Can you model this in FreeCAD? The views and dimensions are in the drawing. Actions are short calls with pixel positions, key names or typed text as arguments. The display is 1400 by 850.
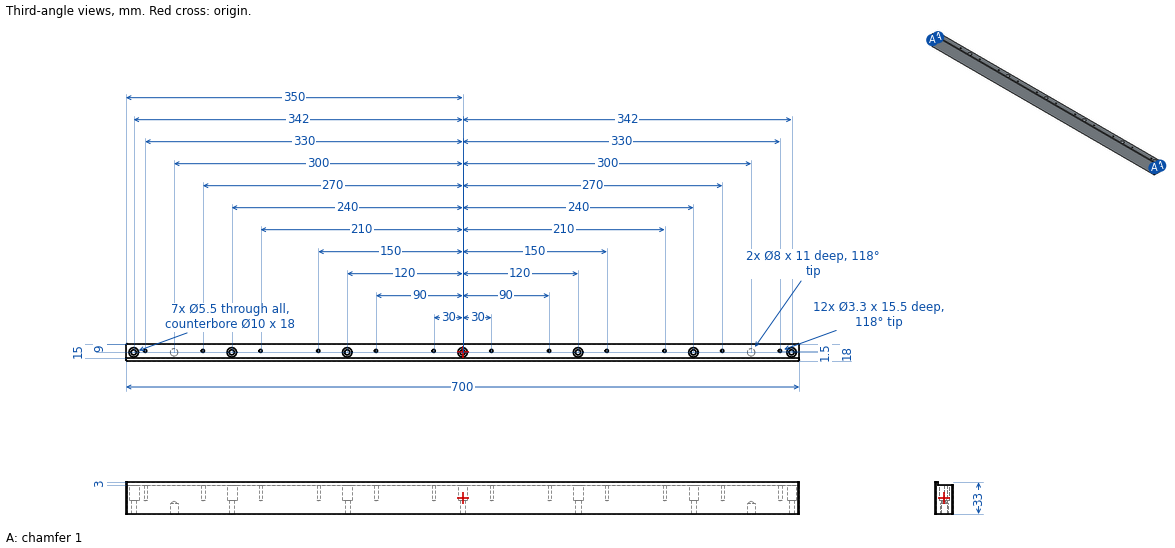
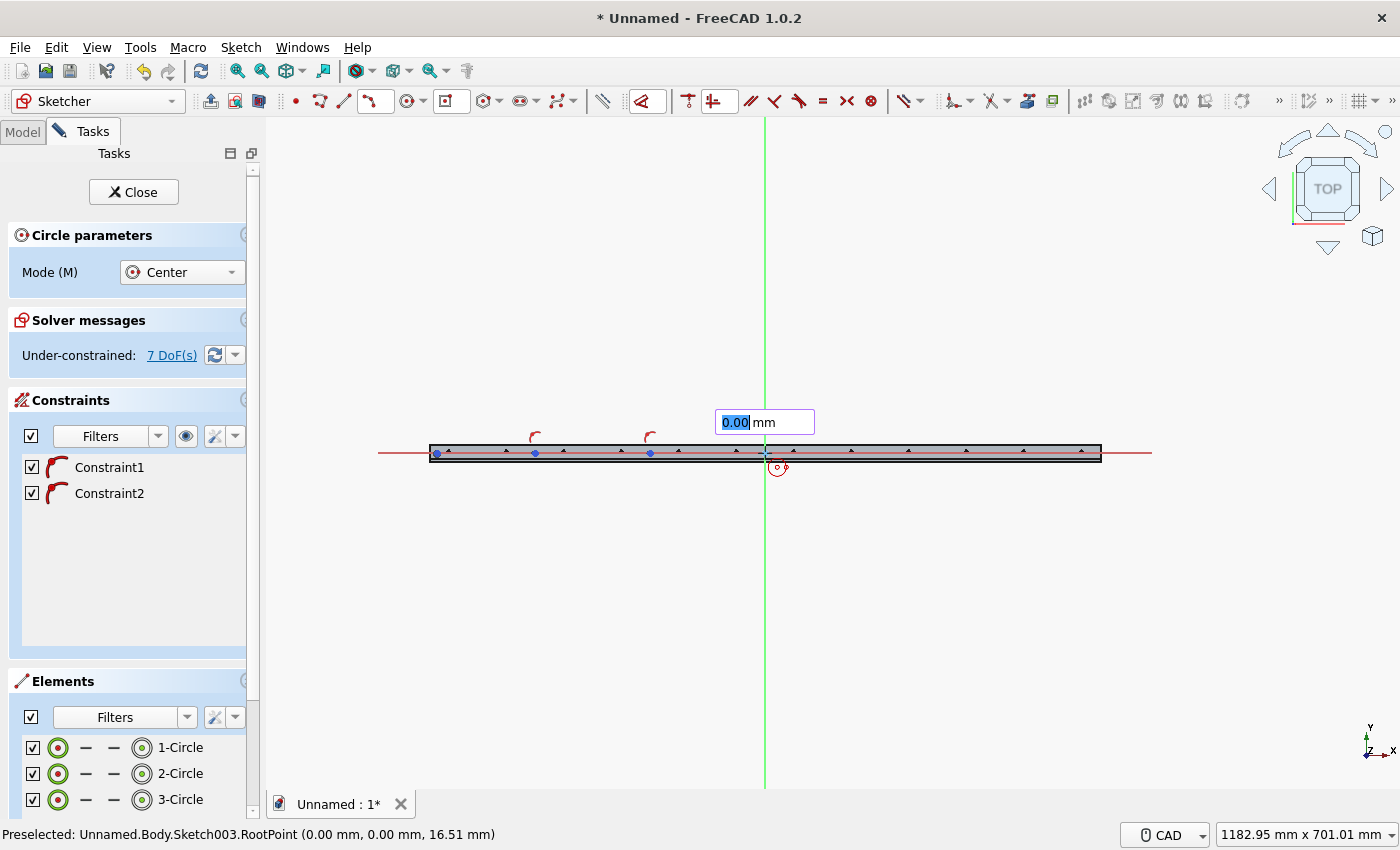
scroll(767, 451, up, 11)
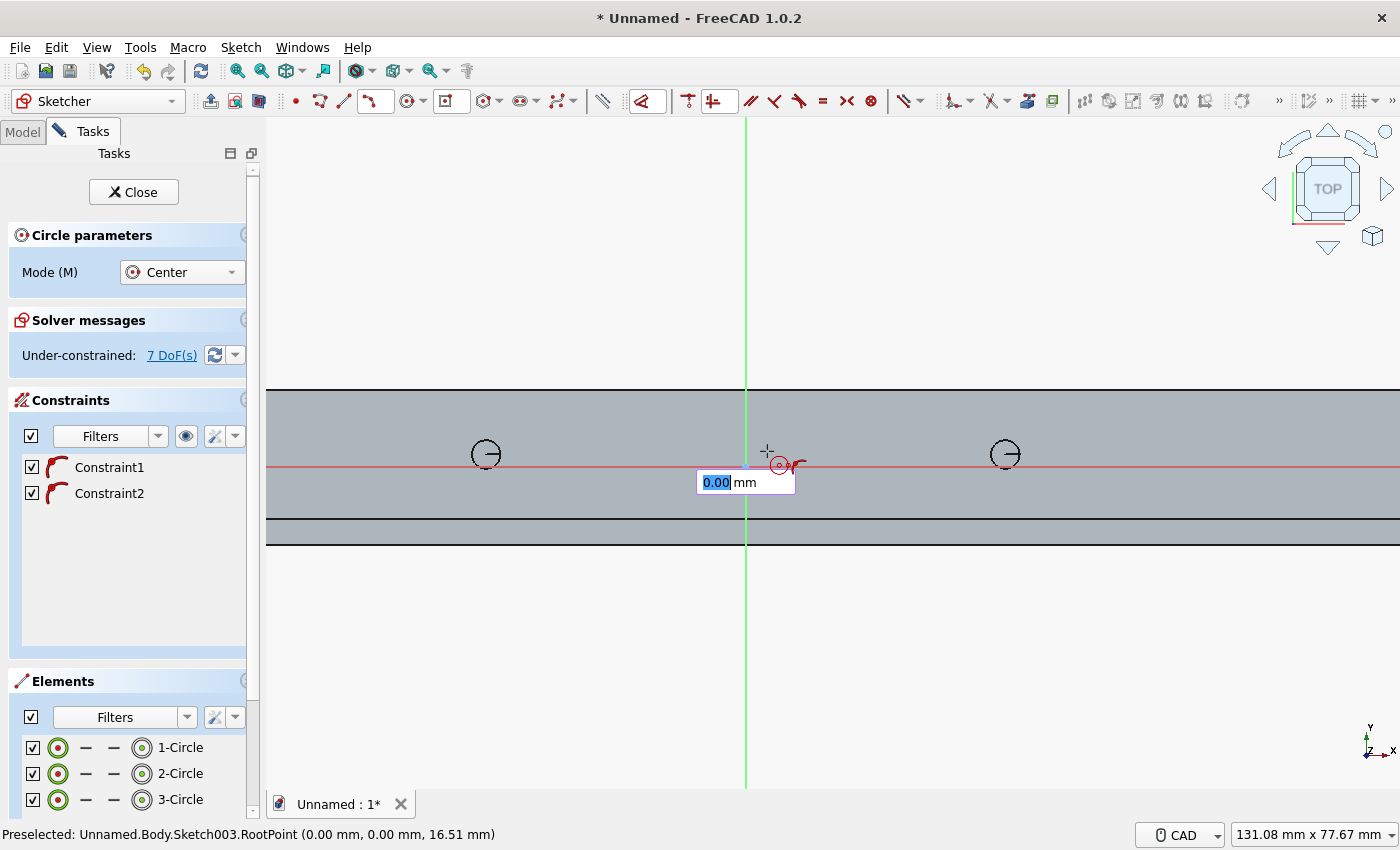
click(763, 451)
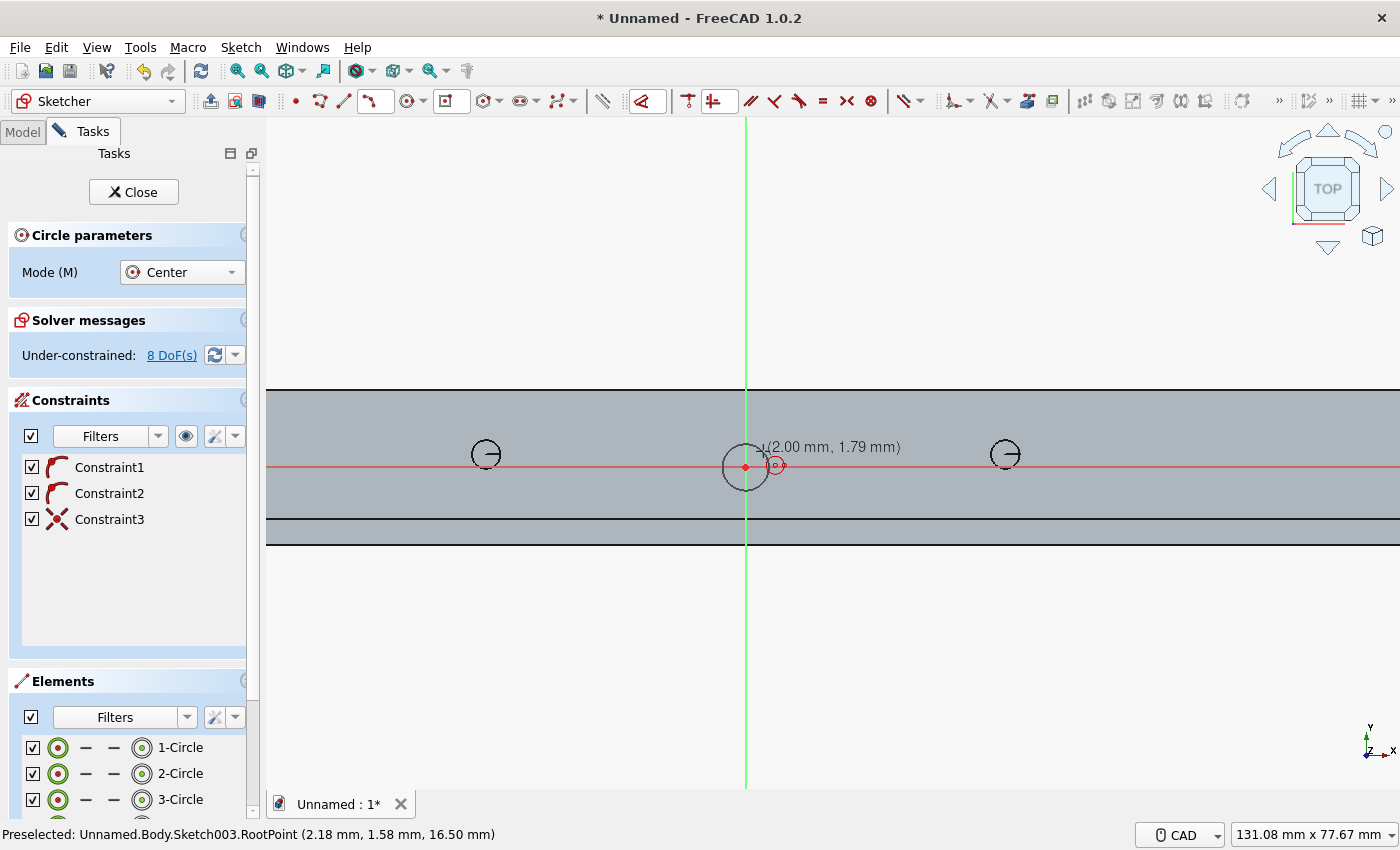
scroll(767, 451, down, 11)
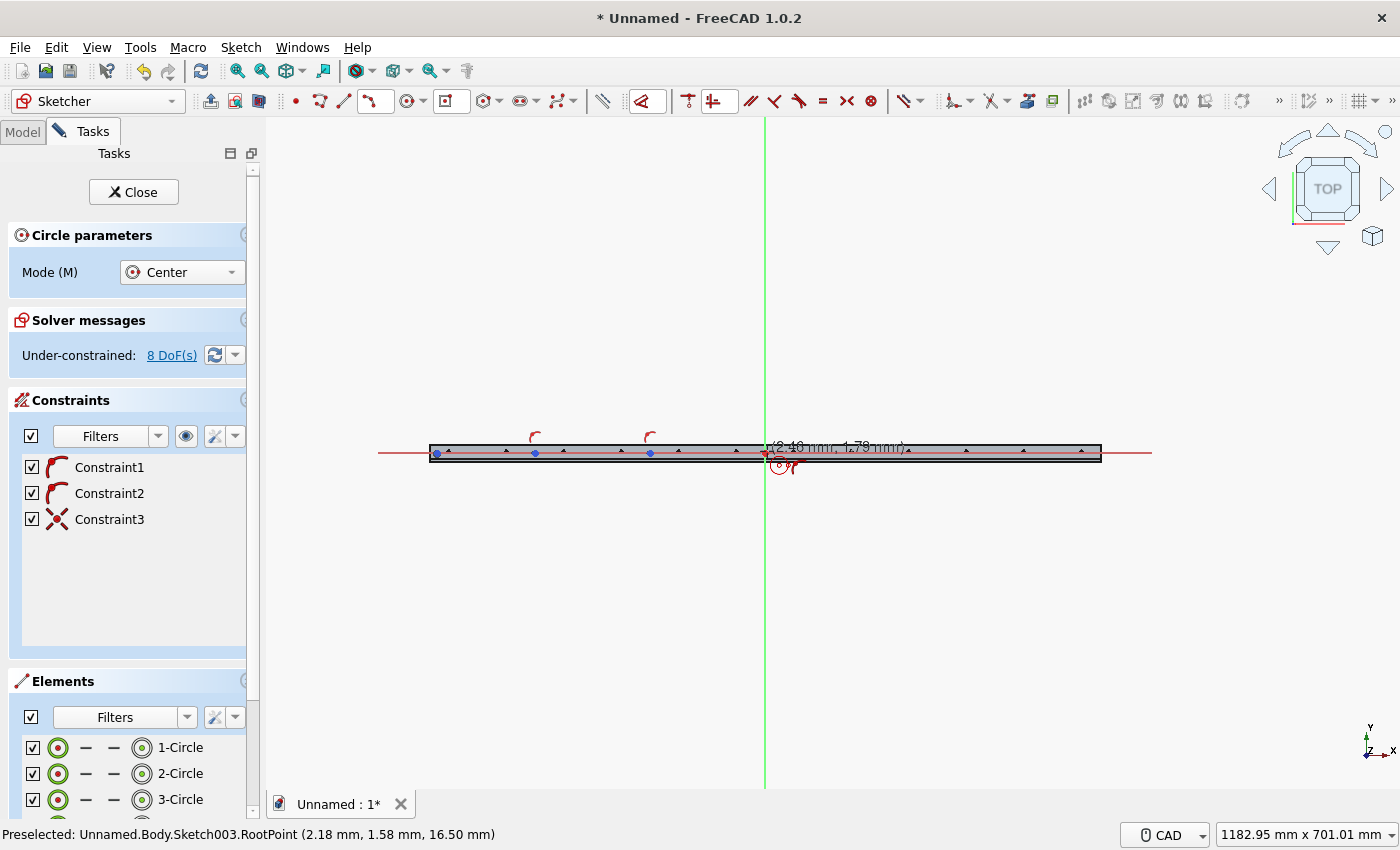
scroll(880, 453, up, 11)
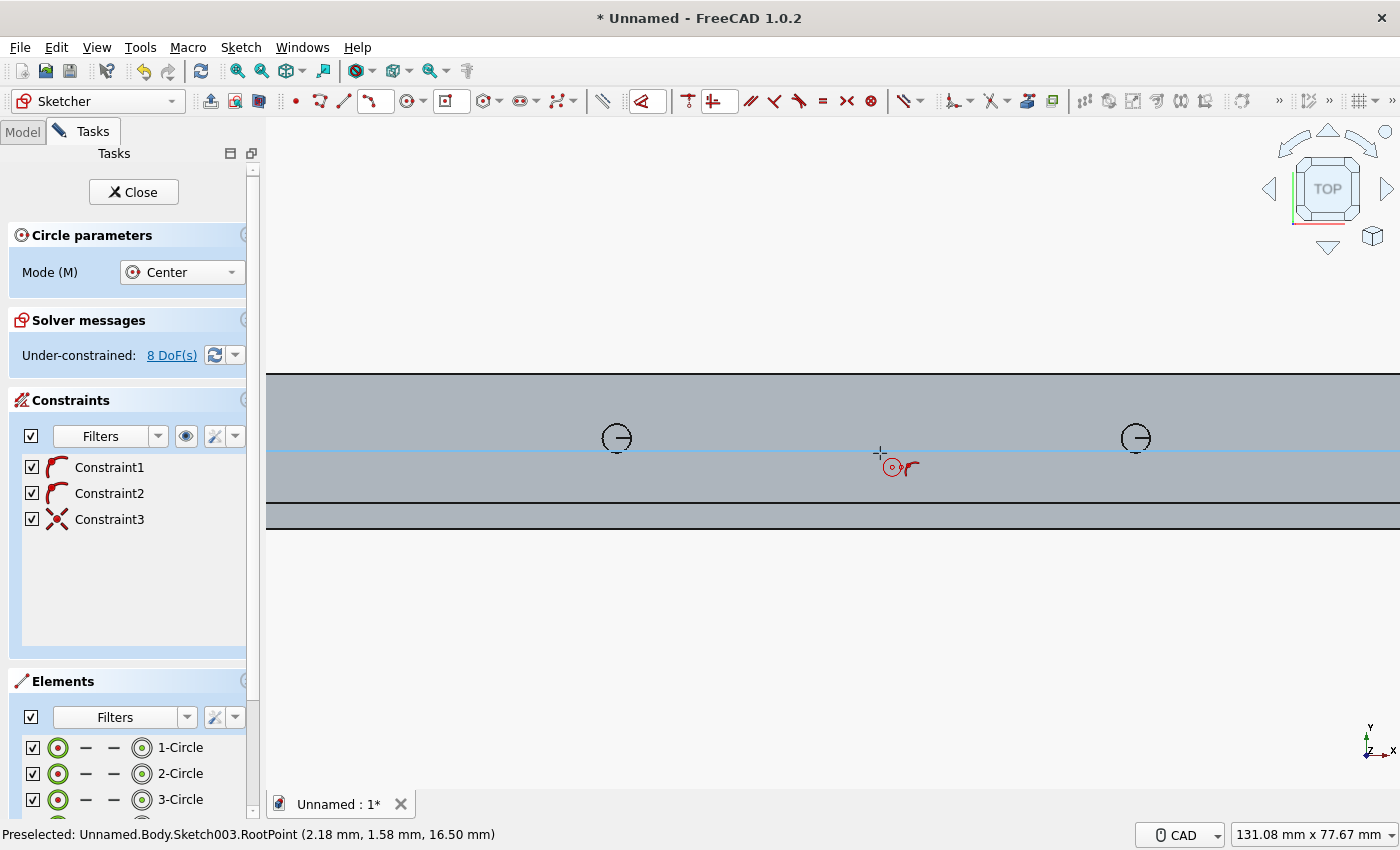
scroll(880, 453, down, 11)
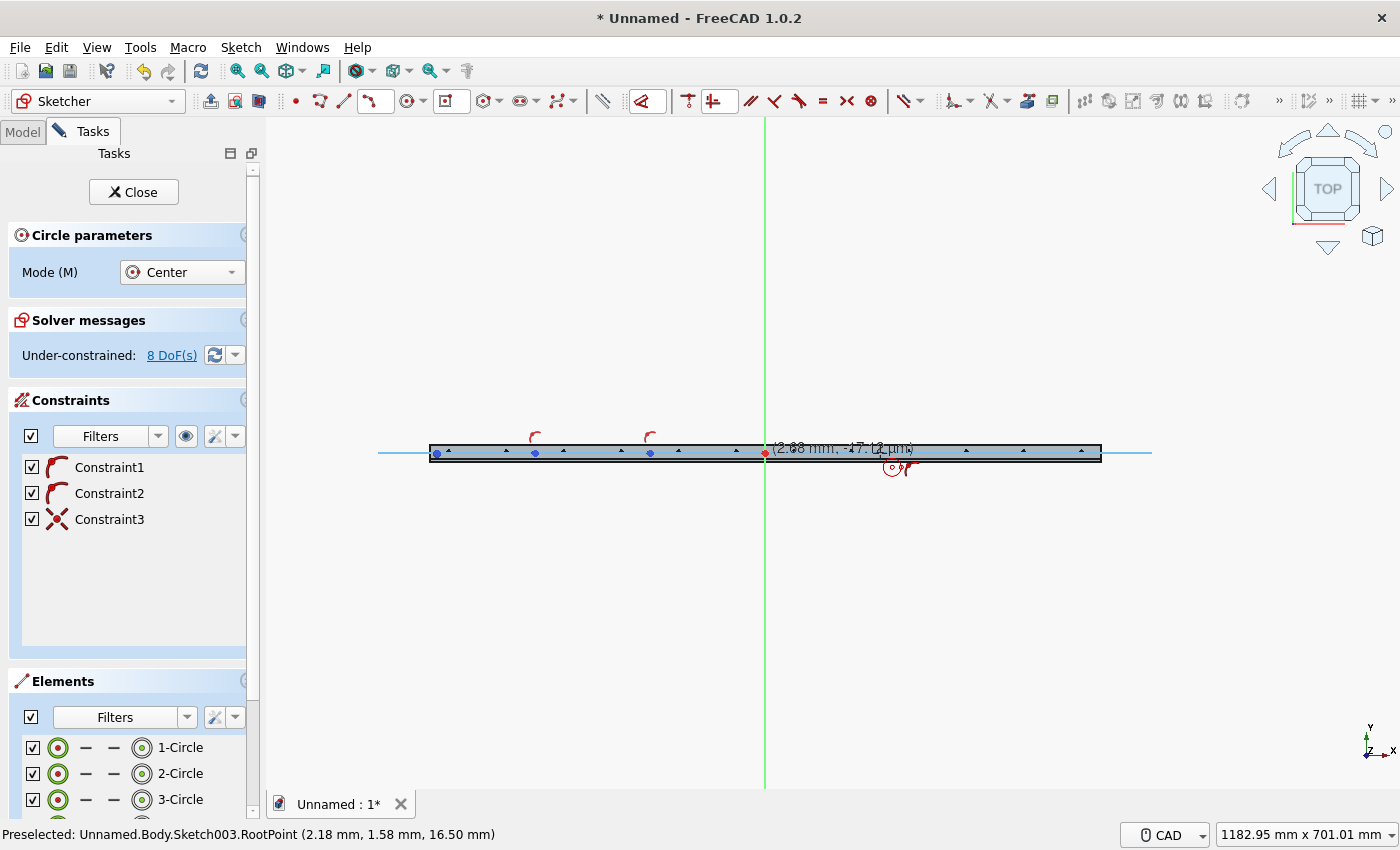
click(880, 453)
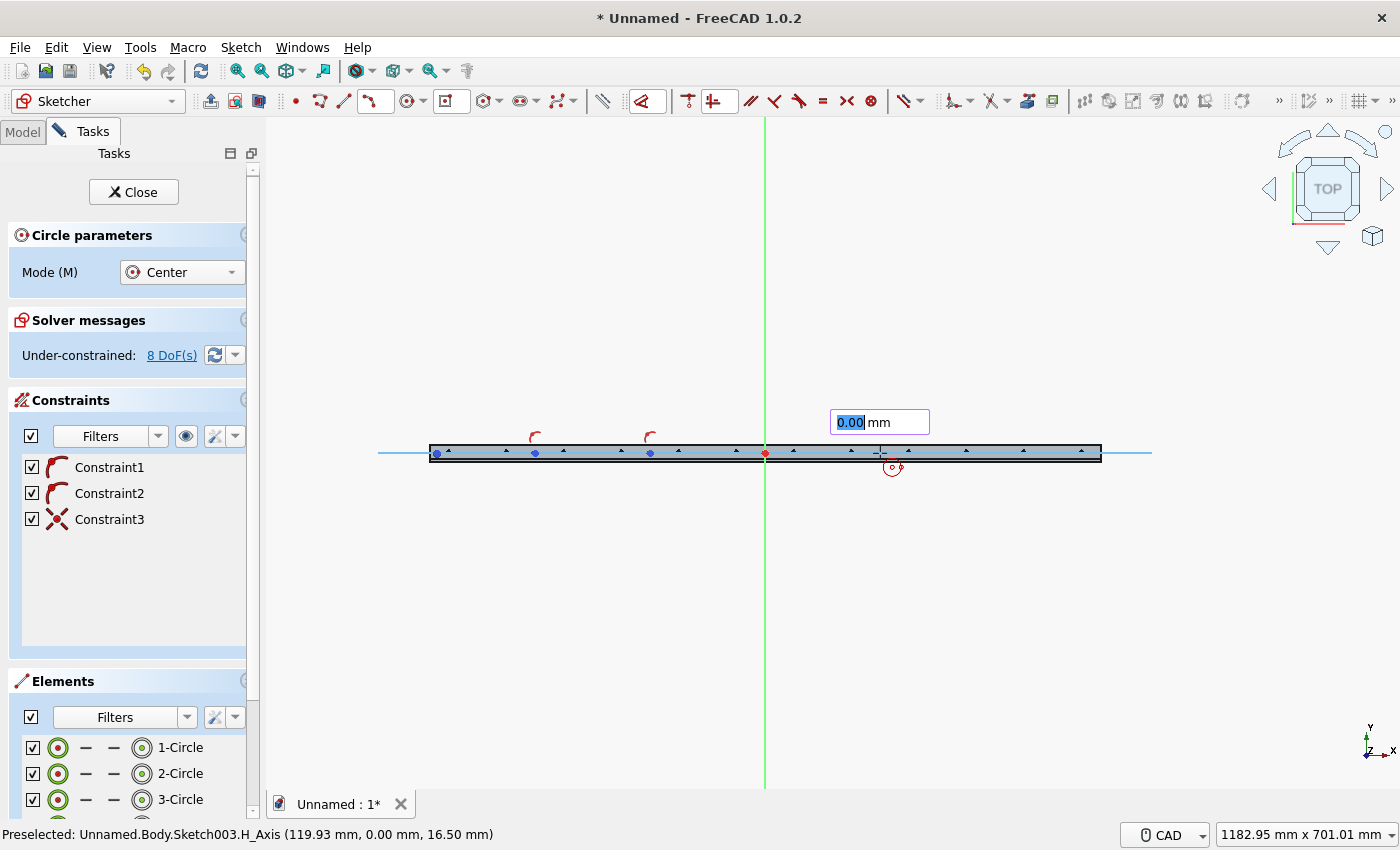
scroll(881, 451, up, 10)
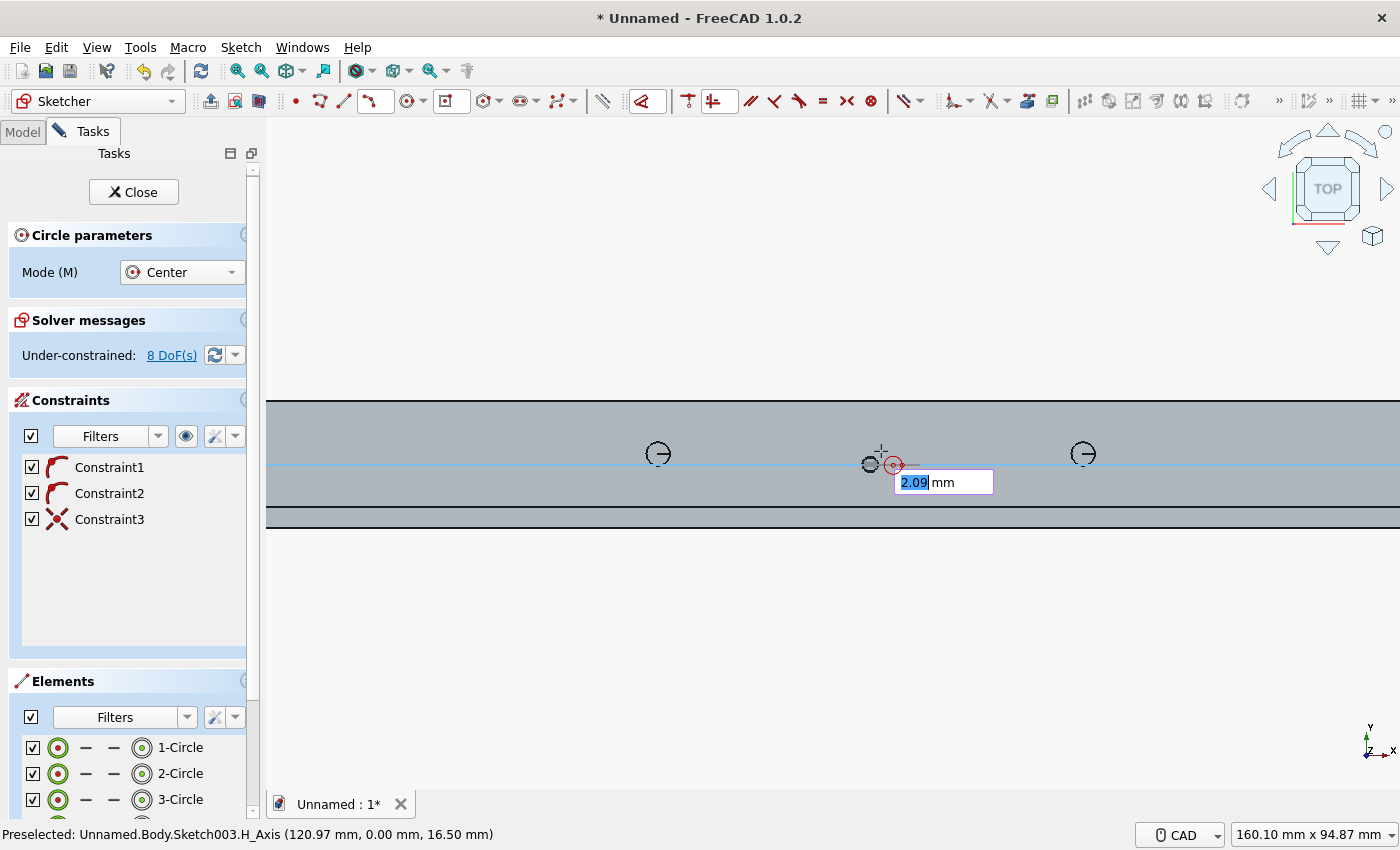
click(877, 446)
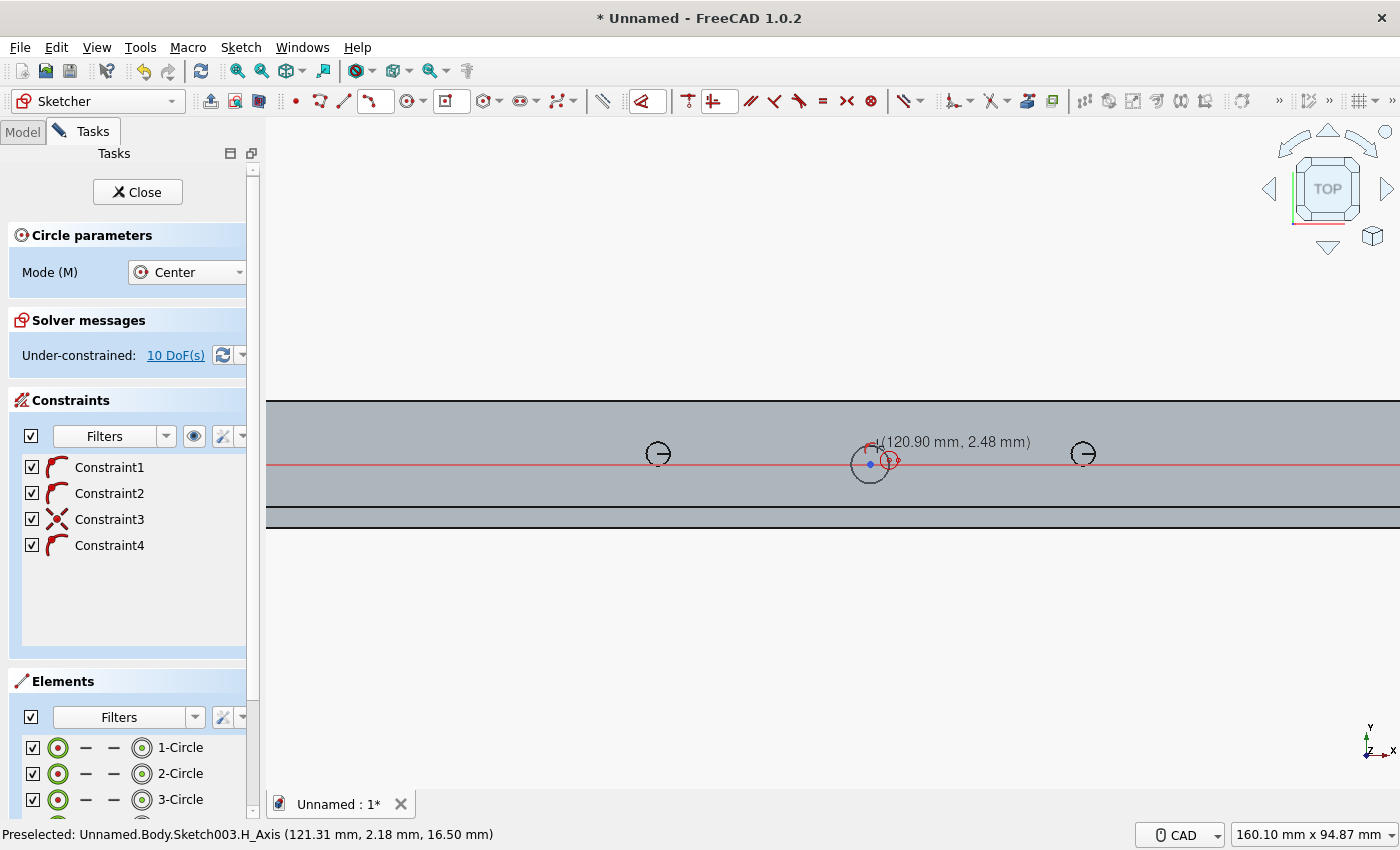
scroll(881, 451, down, 10)